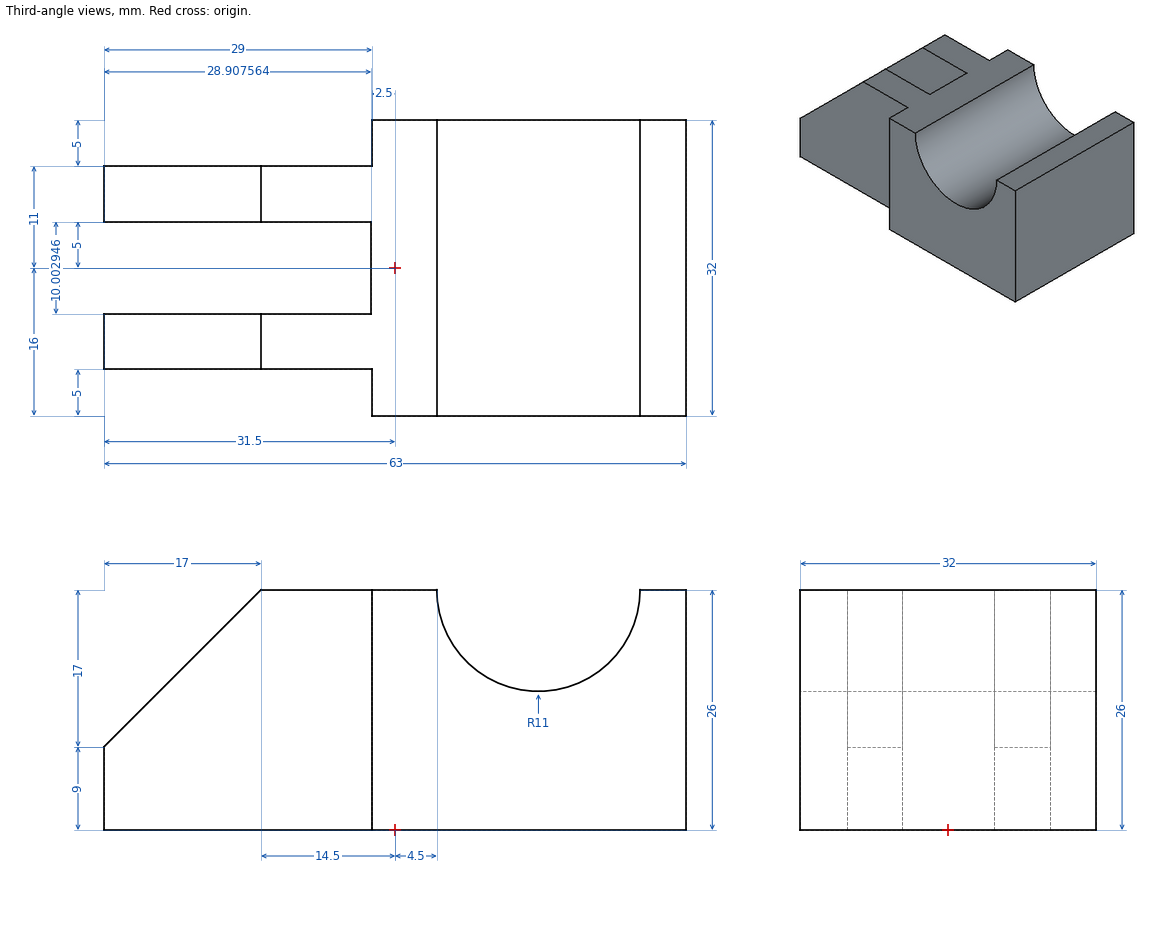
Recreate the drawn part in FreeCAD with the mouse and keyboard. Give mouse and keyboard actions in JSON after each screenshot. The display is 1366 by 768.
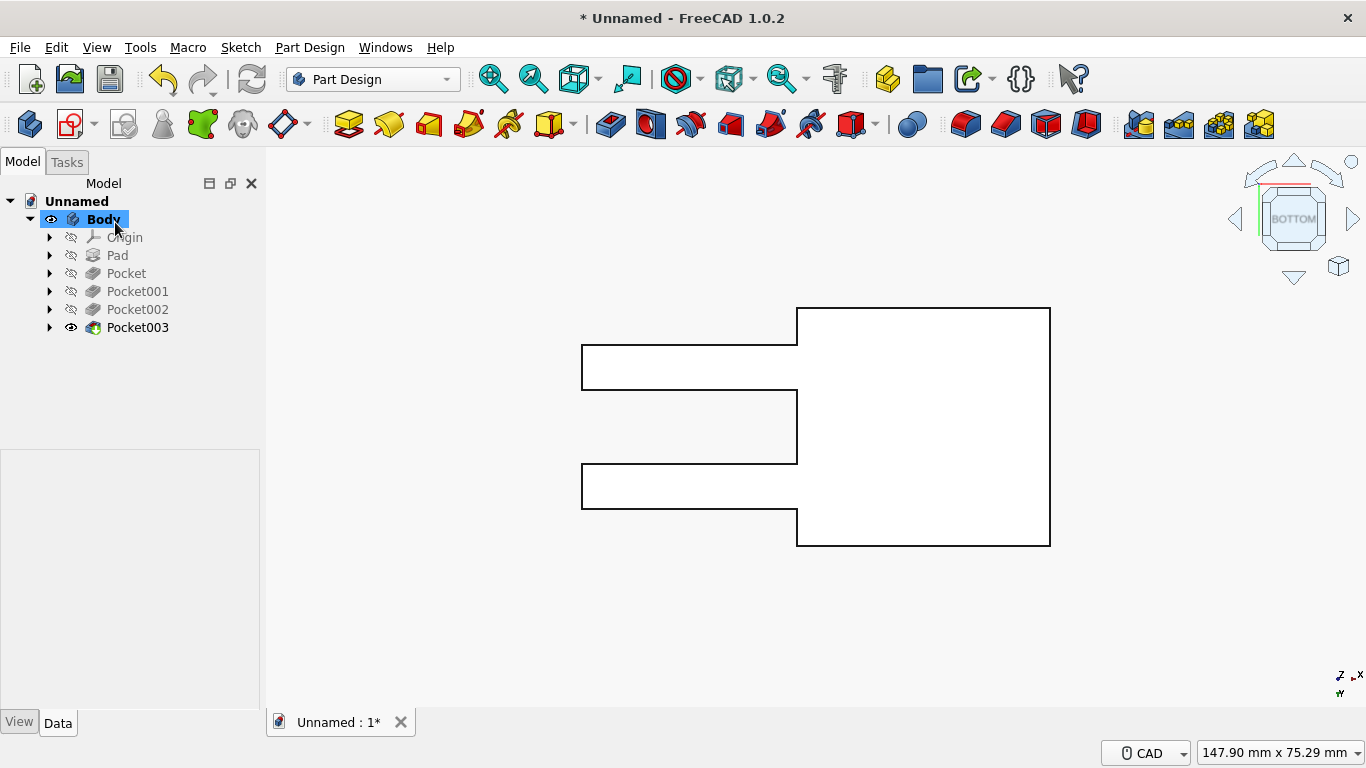
{"action": "key", "text": "0"}